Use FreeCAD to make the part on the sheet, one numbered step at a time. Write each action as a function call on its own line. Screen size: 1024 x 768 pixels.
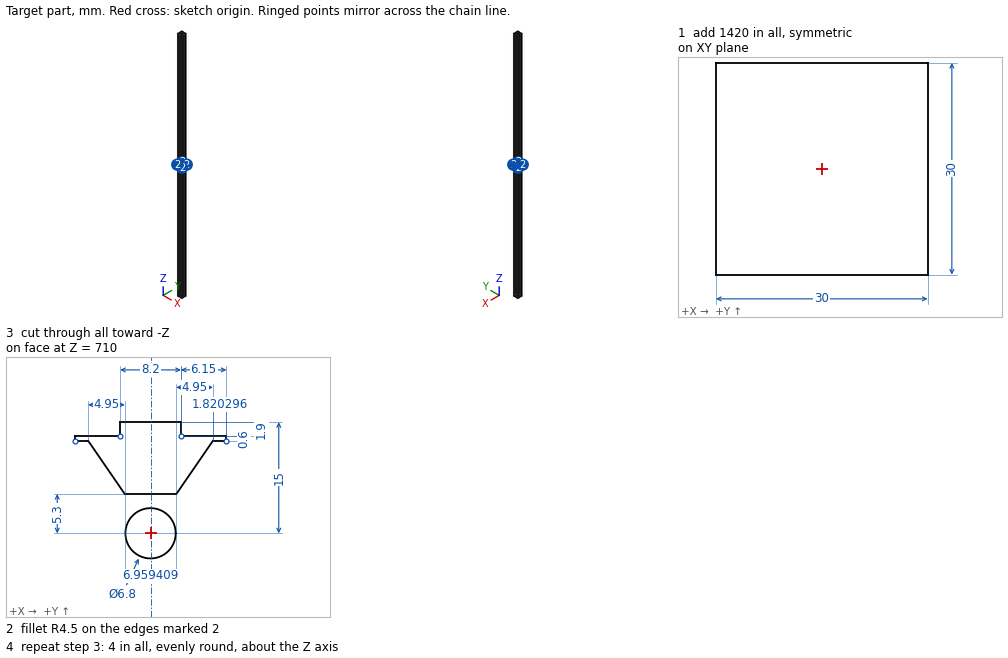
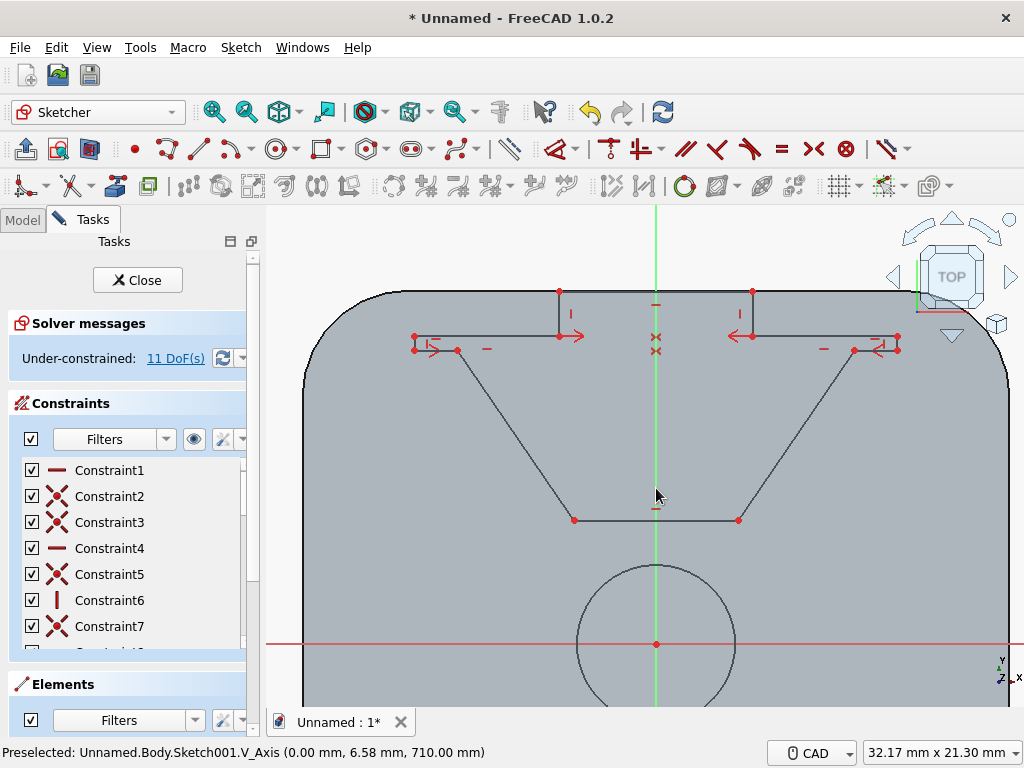
click(712, 588)
click(735, 565)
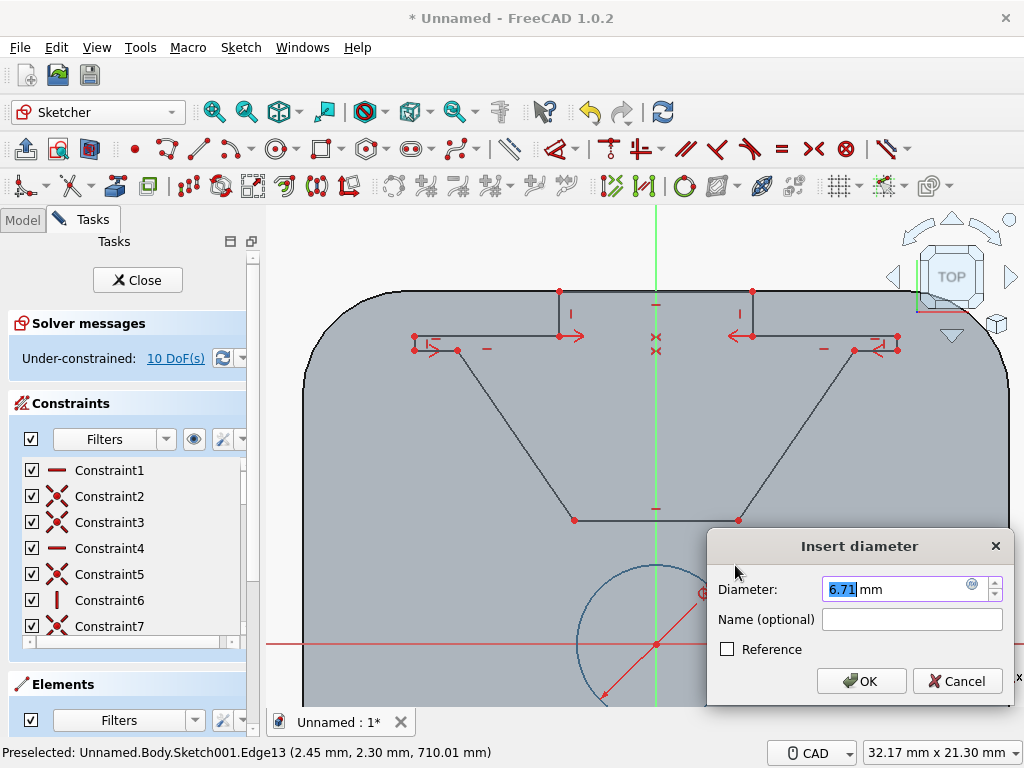
text(6.8)
key(Return)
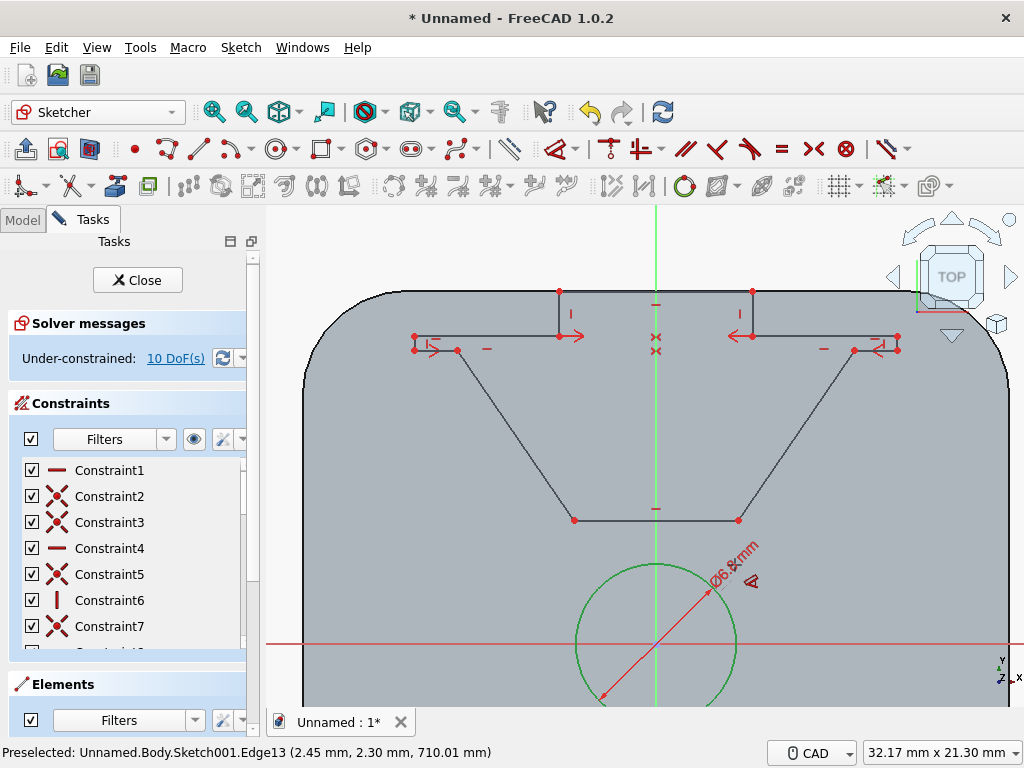
scroll(415, 351, down, 2)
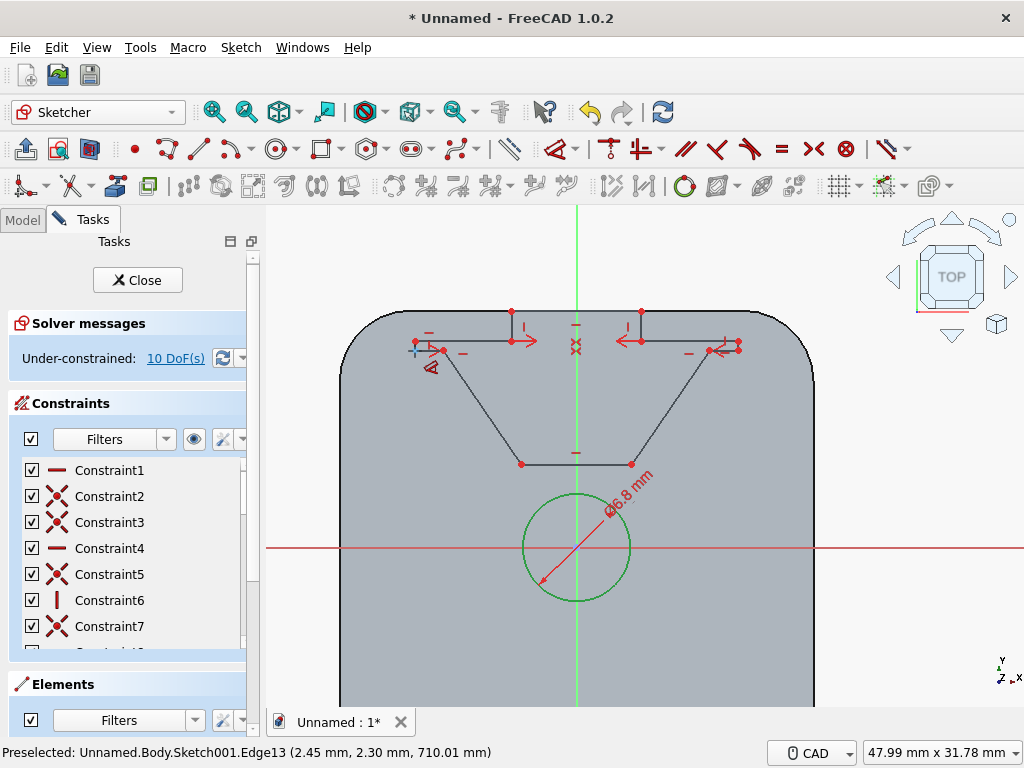
scroll(738, 346, up, 8)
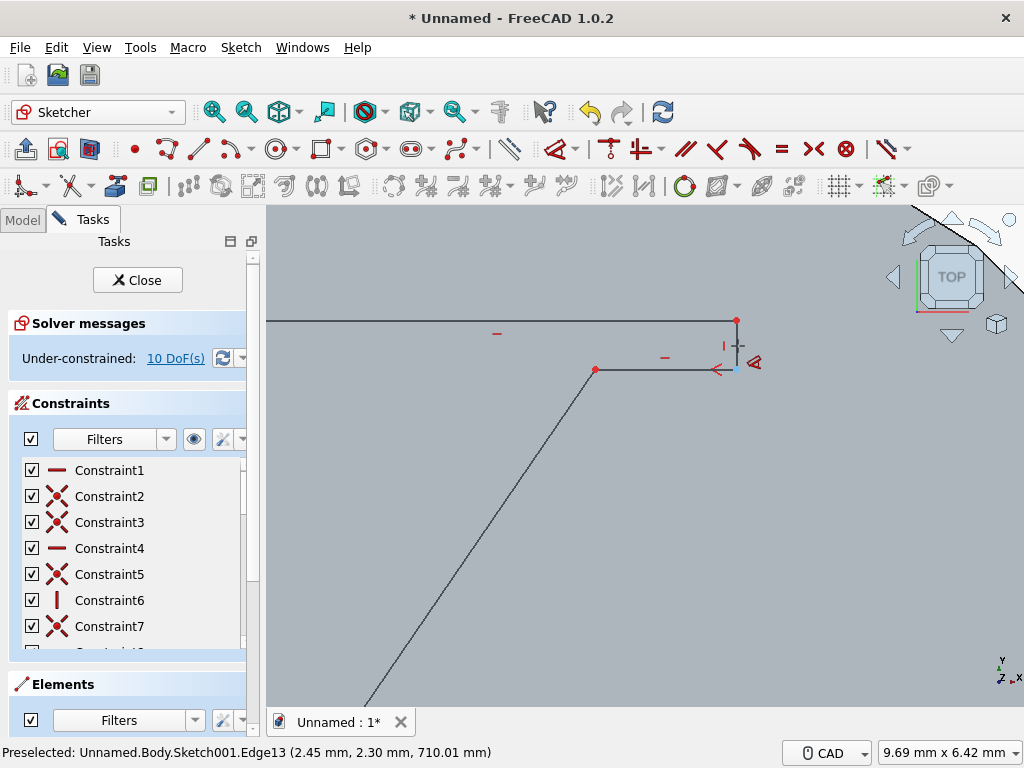
click(737, 345)
click(771, 345)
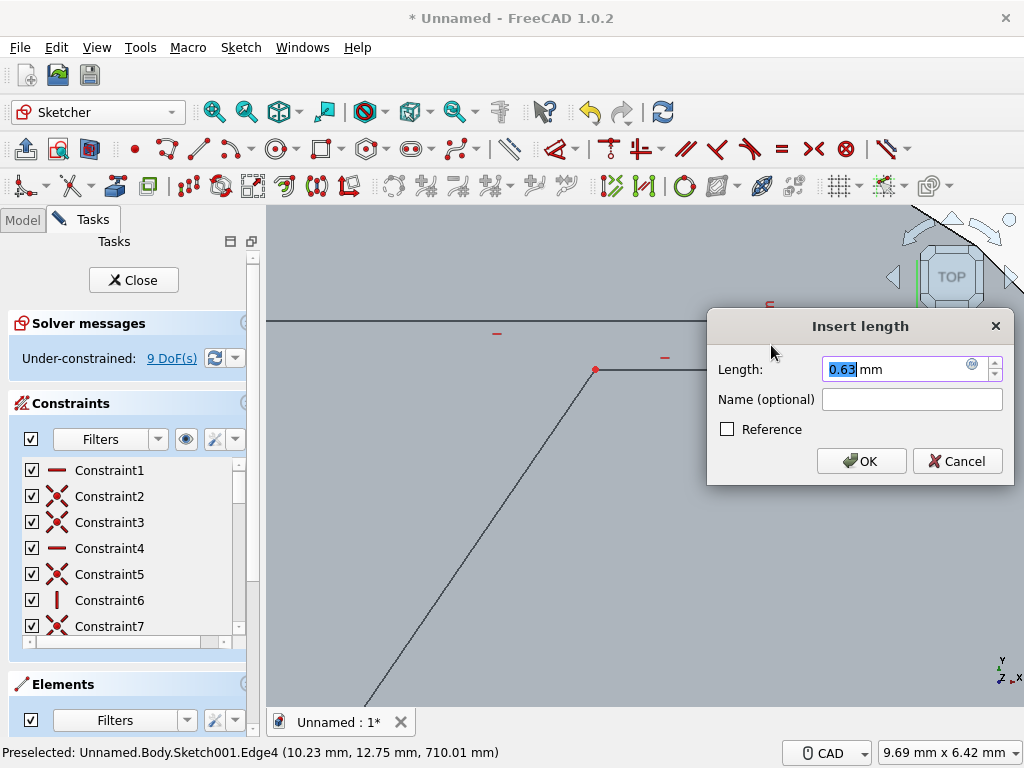
text(0.6)
key(Return)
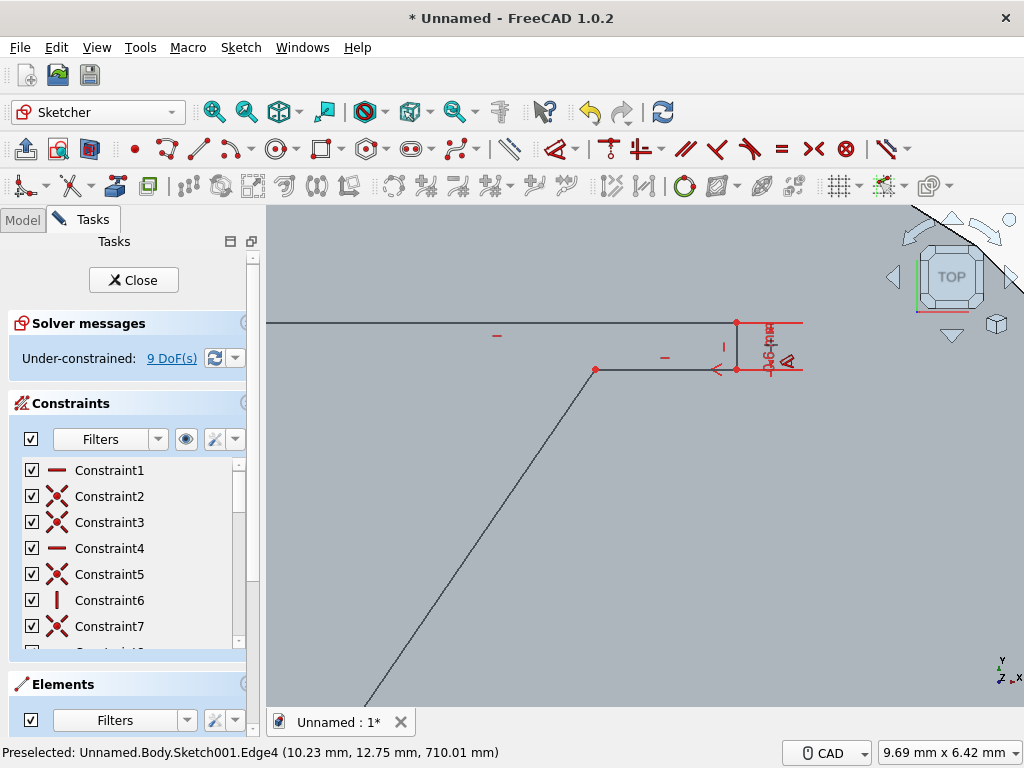
scroll(738, 346, down, 8)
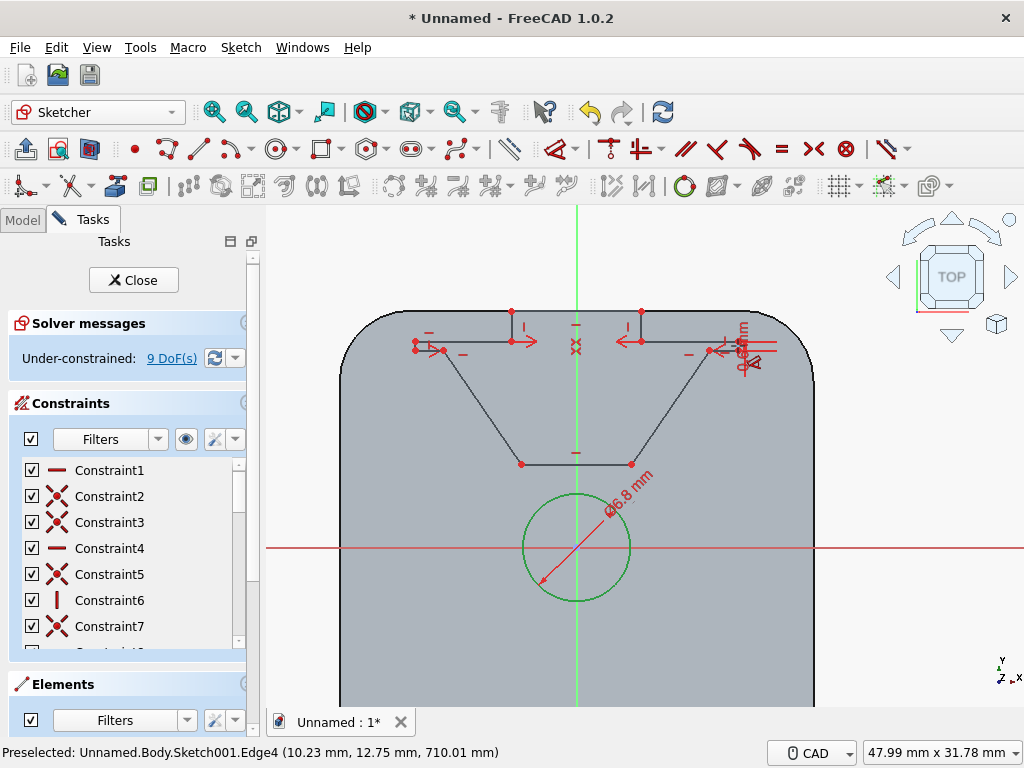
scroll(641, 332, up, 3)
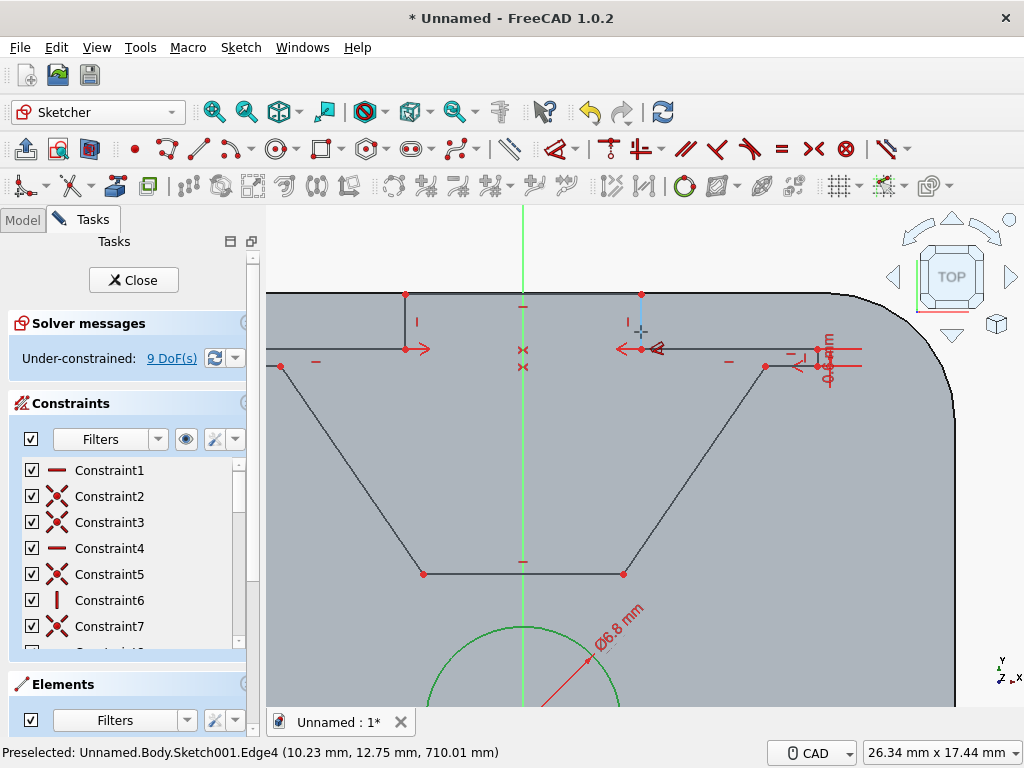
click(641, 333)
click(675, 322)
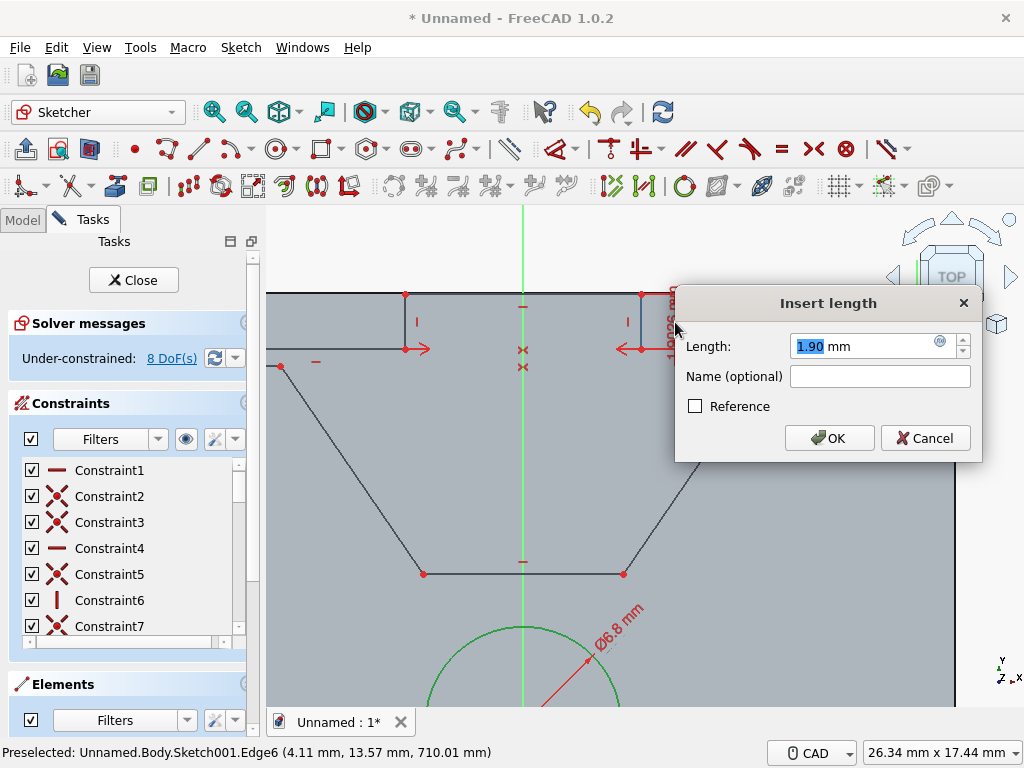
text(1.9)
key(Return)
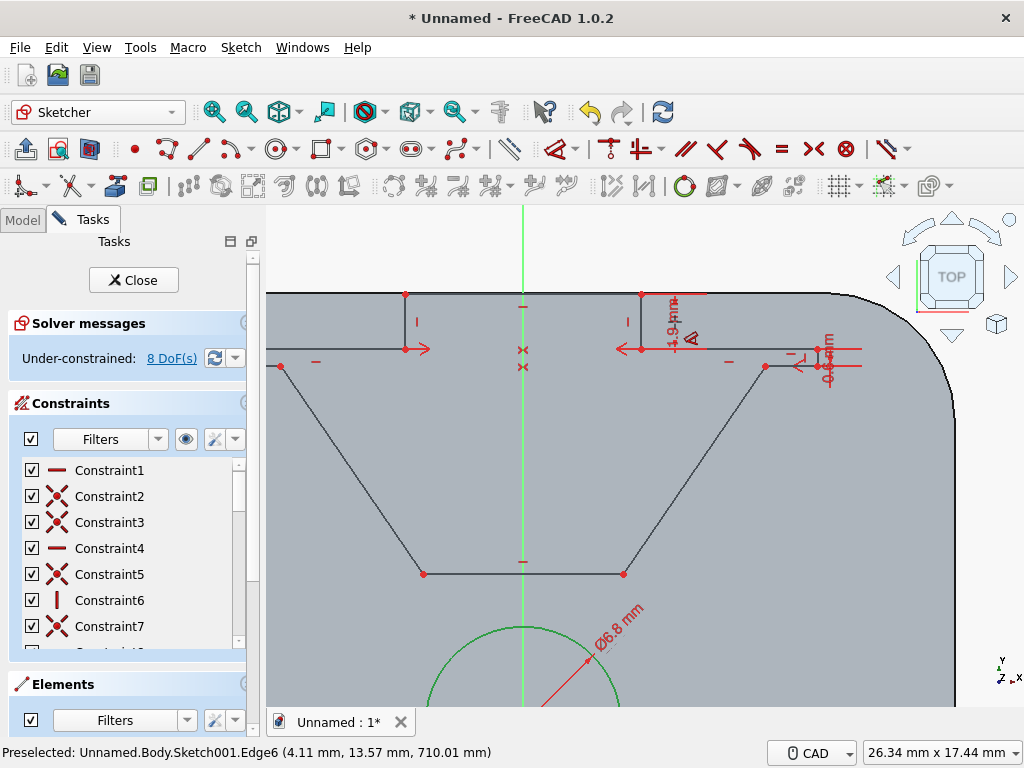
click(571, 294)
click(469, 260)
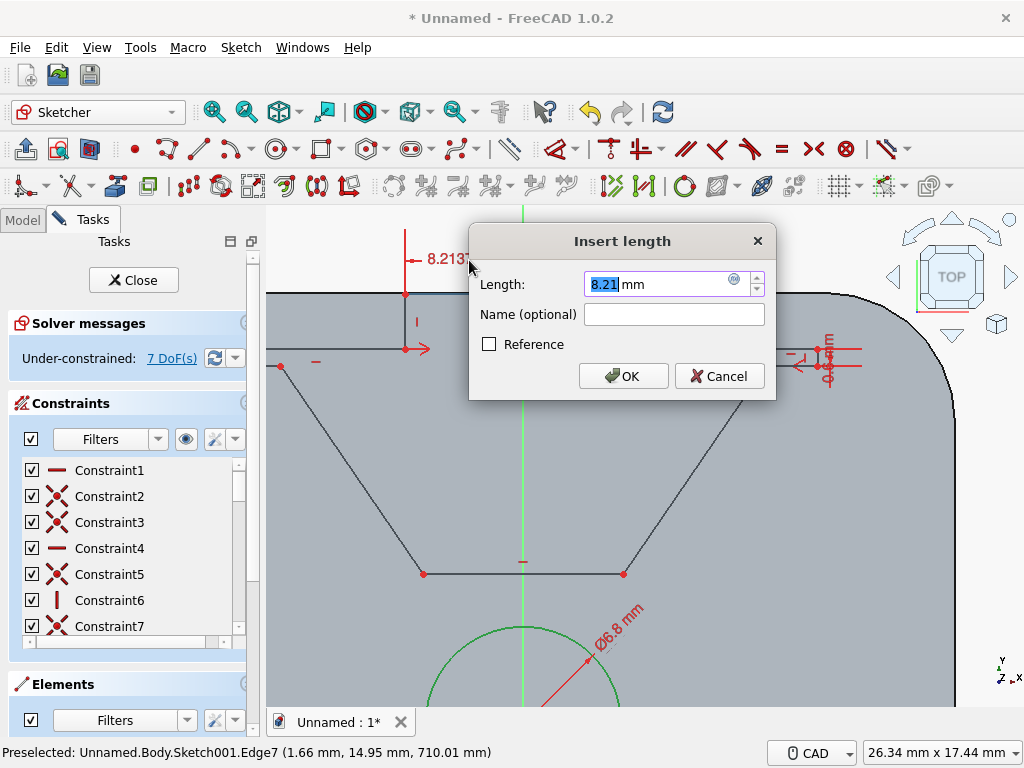
text(8.2)
key(Return)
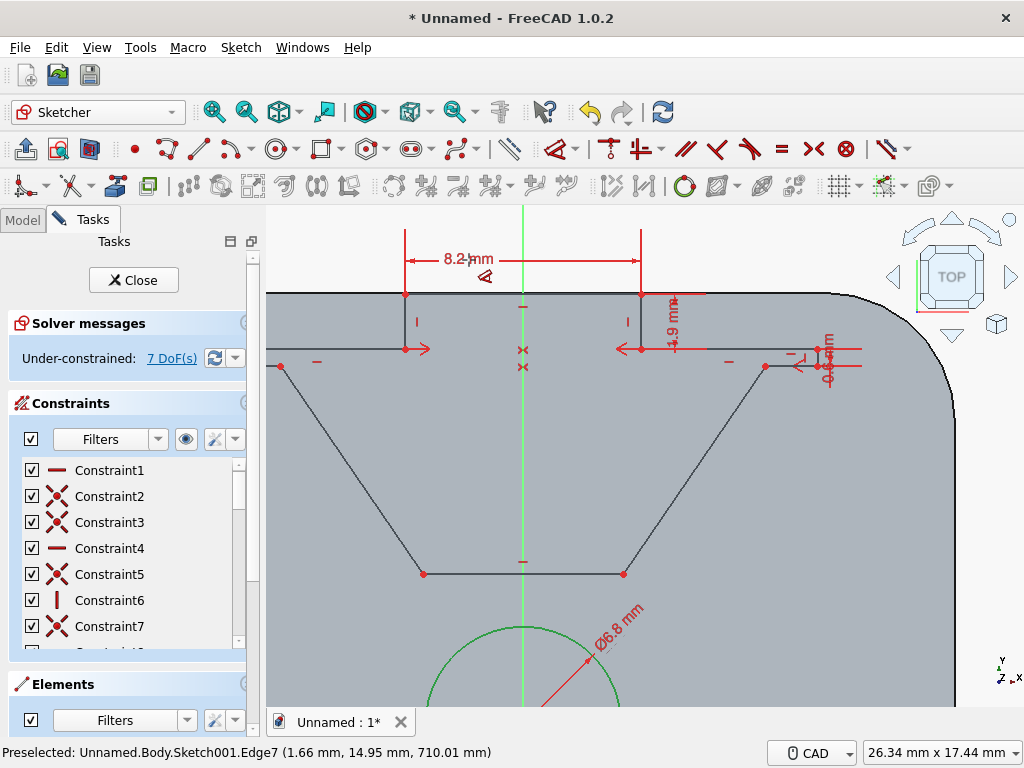
click(641, 294)
click(675, 398)